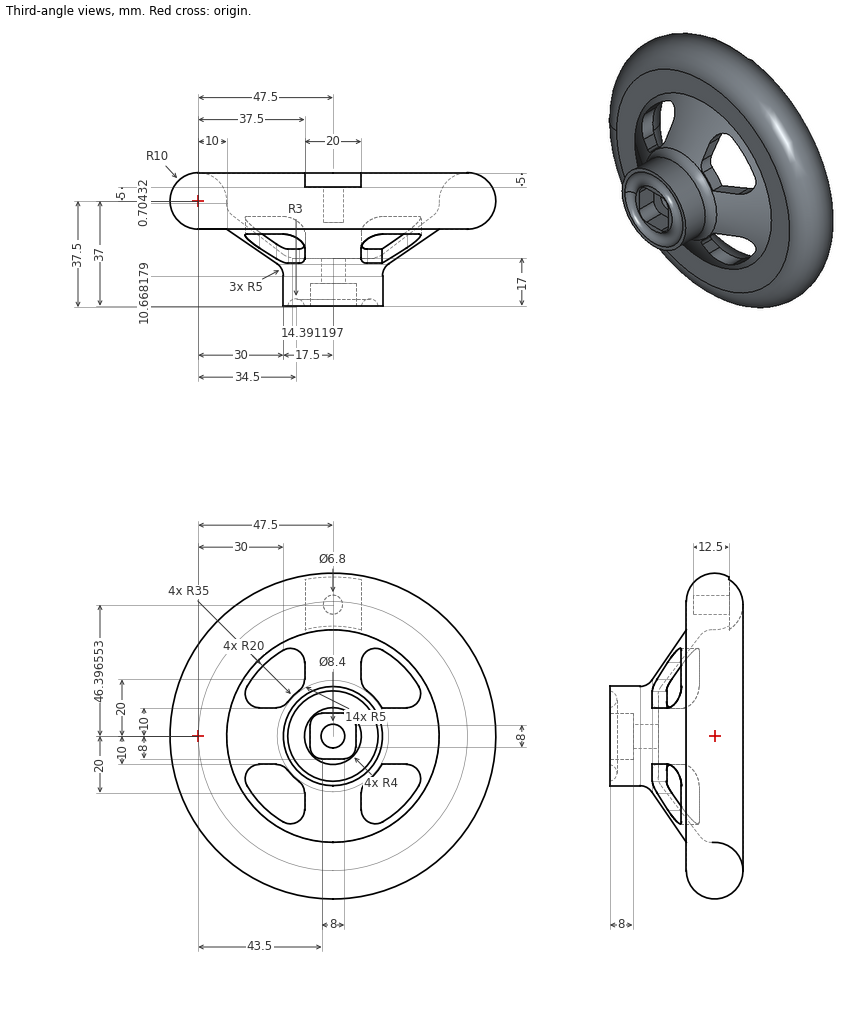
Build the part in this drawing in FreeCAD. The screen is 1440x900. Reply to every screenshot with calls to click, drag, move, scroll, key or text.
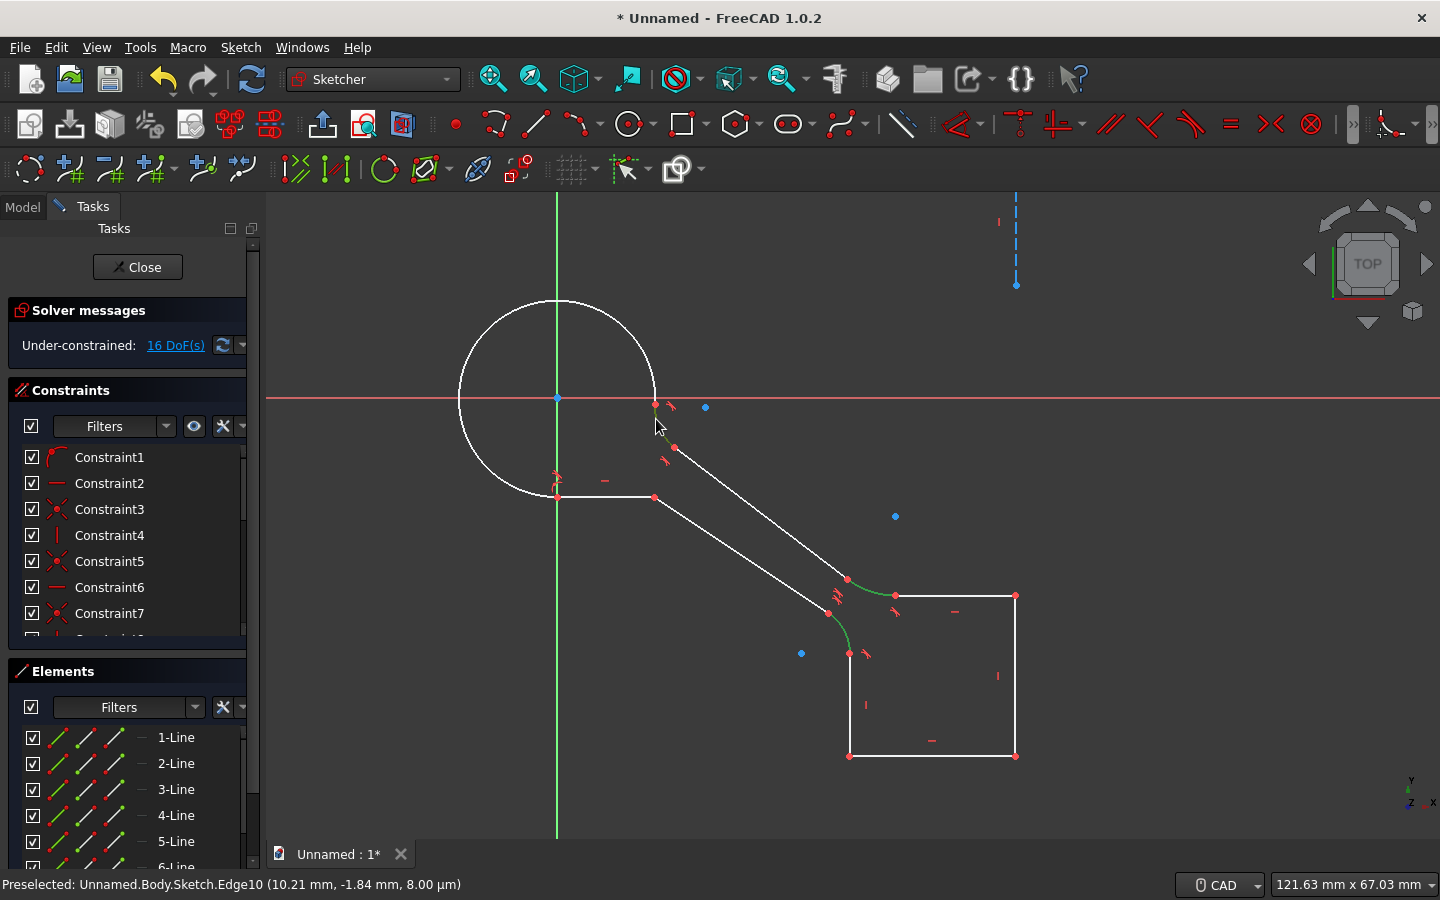
click(1232, 124)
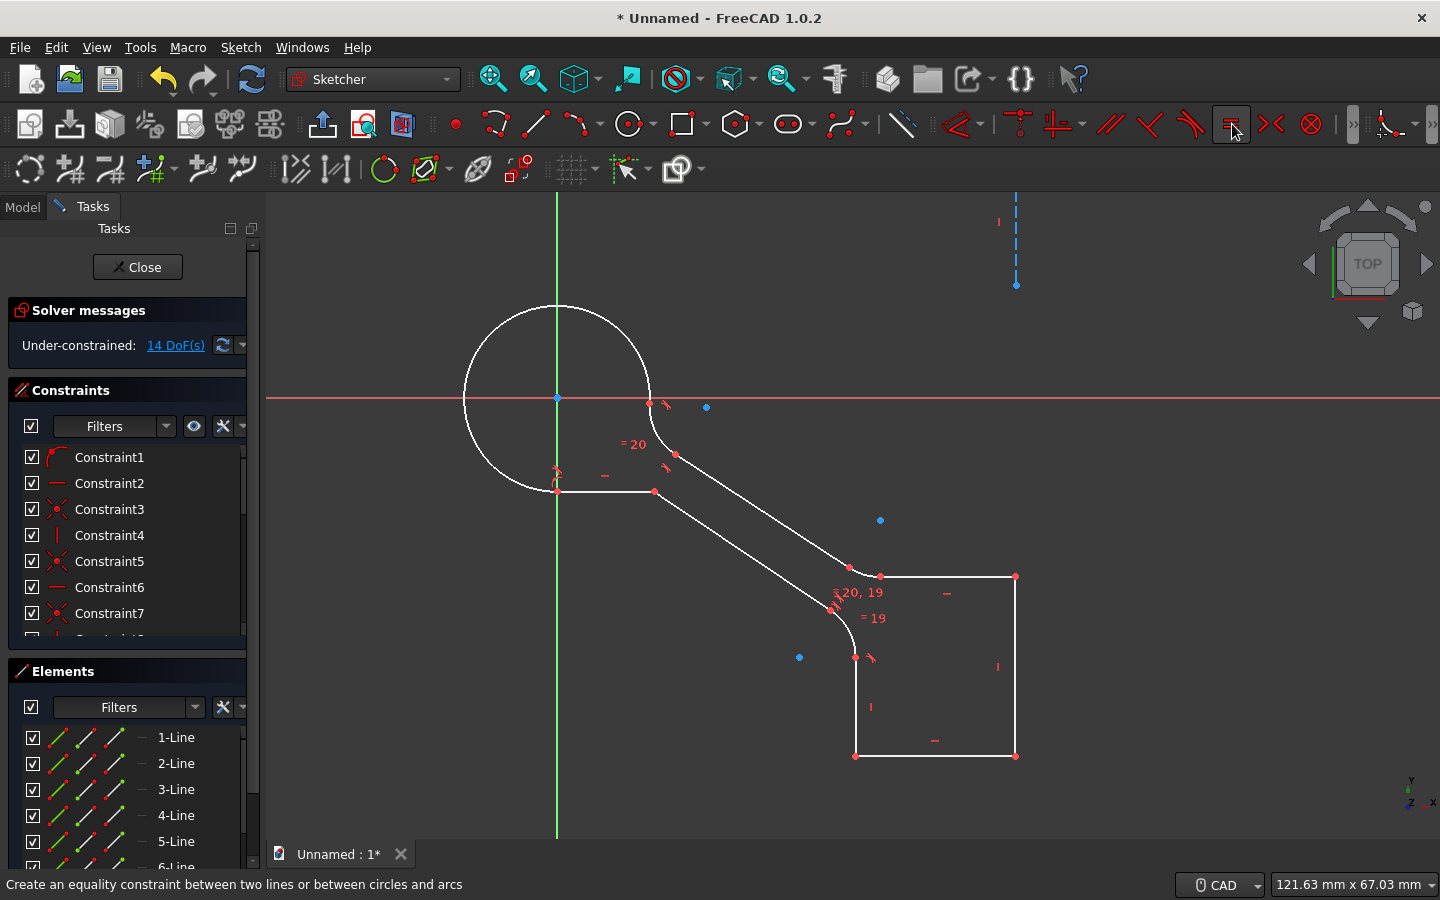
click(557, 399)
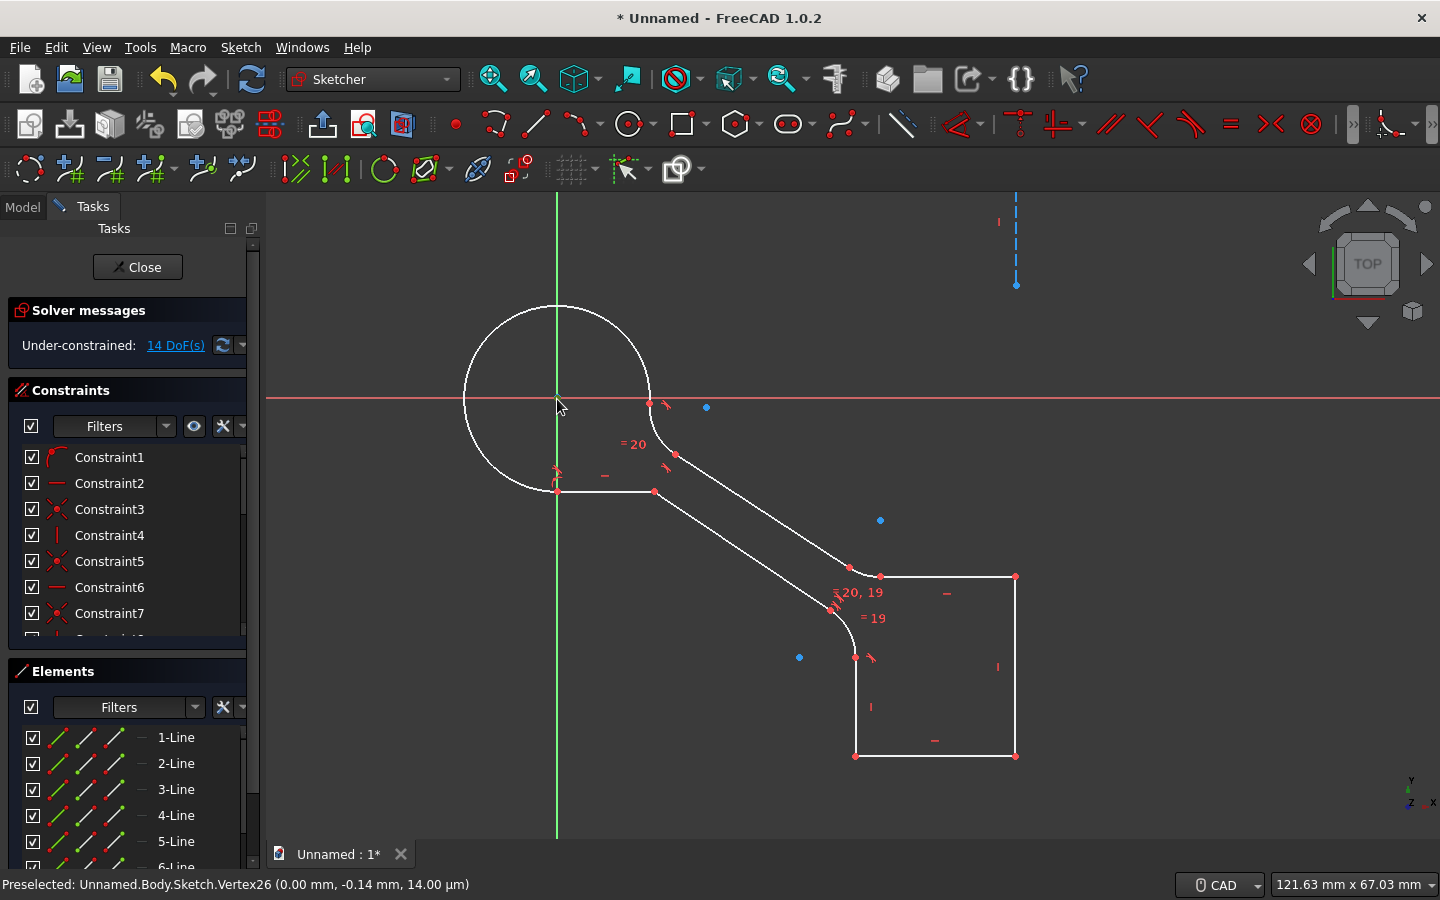
click(364, 398)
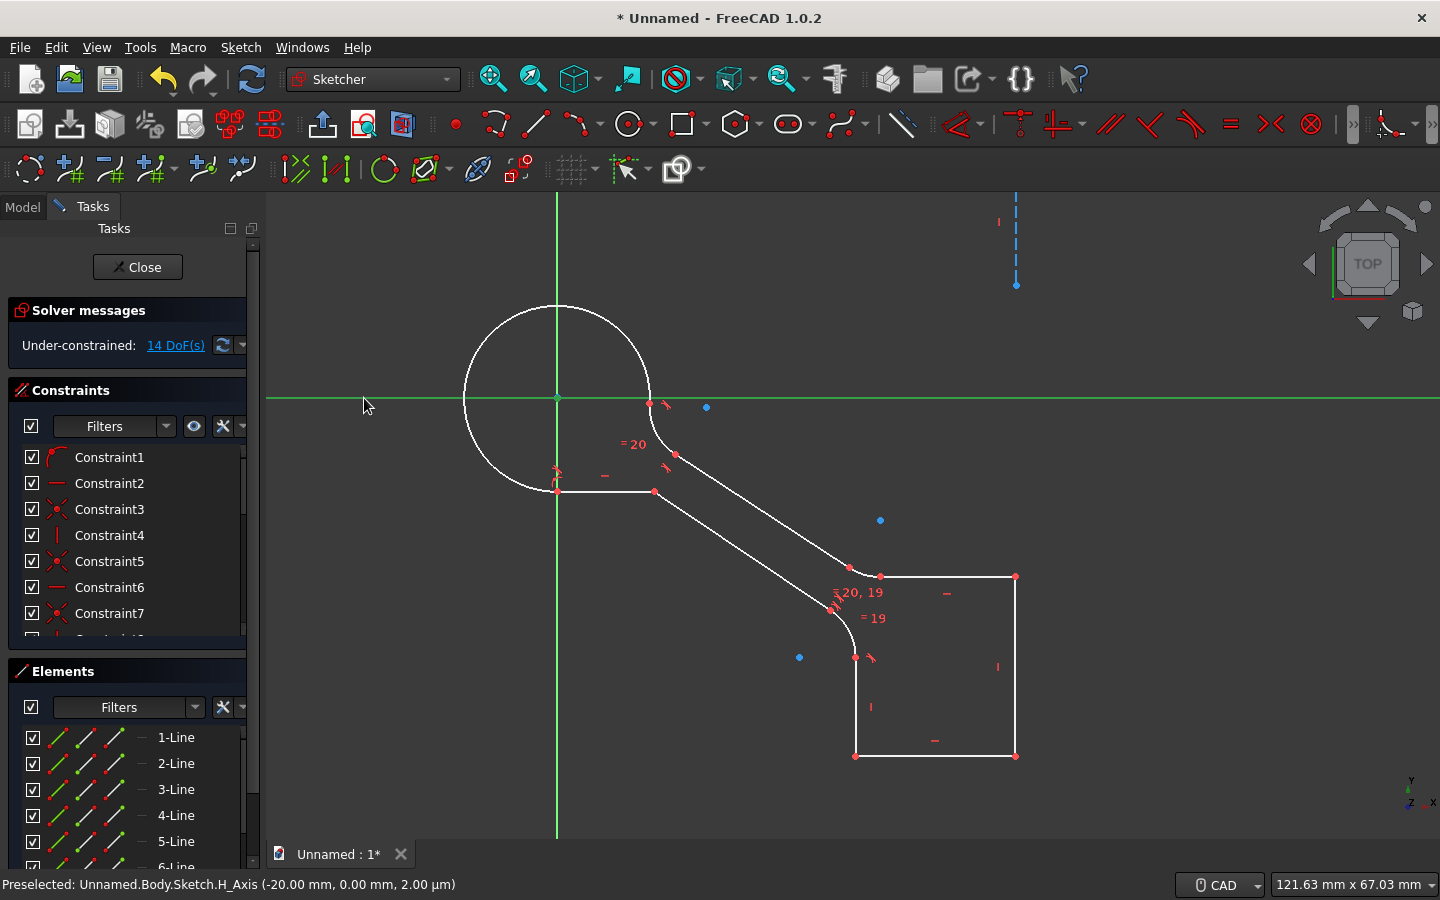
click(1018, 124)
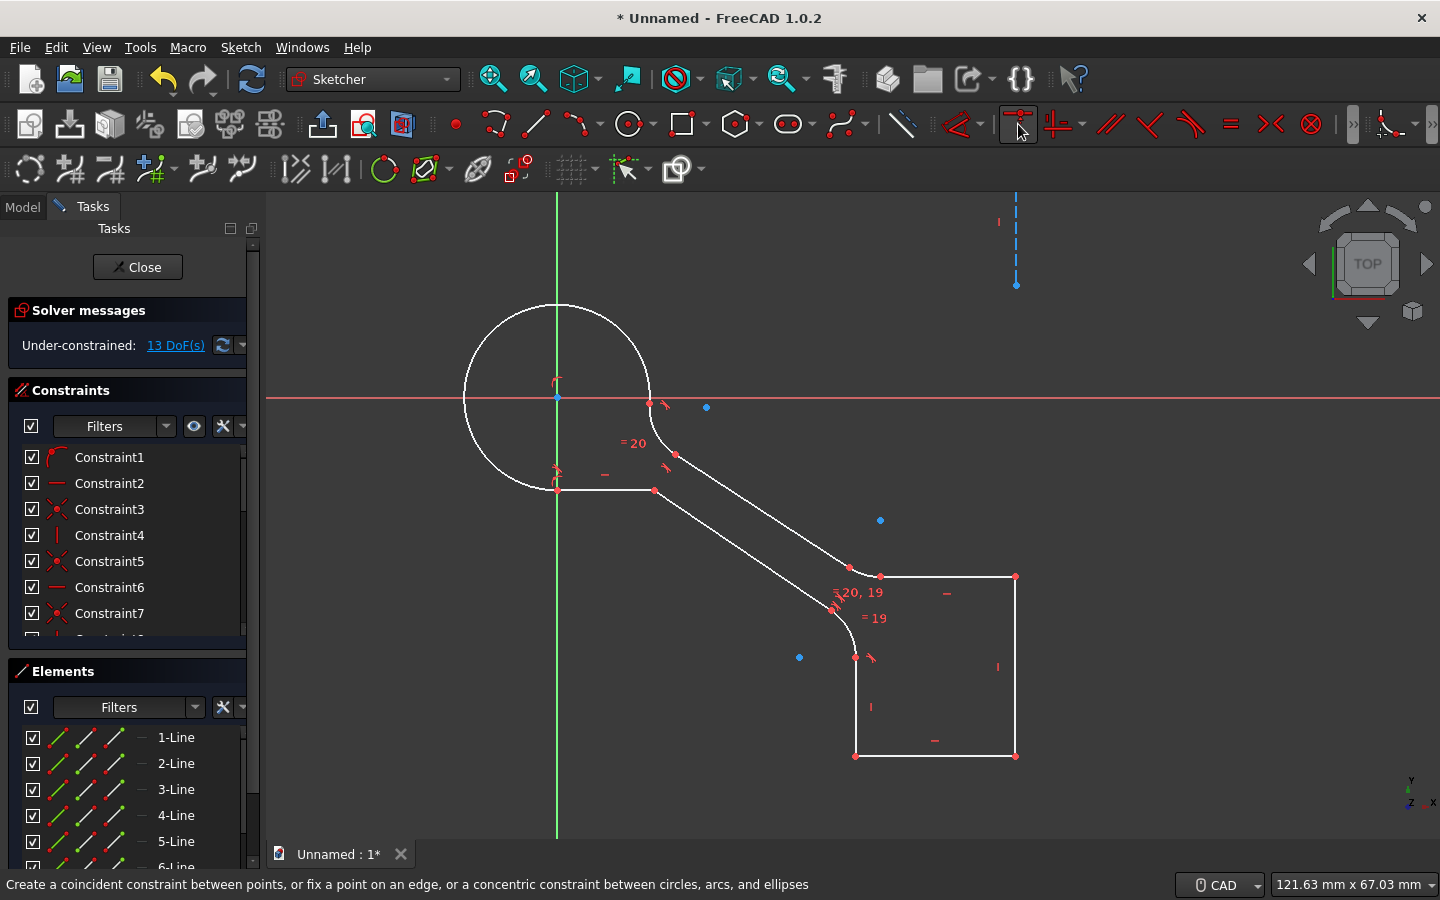
click(956, 124)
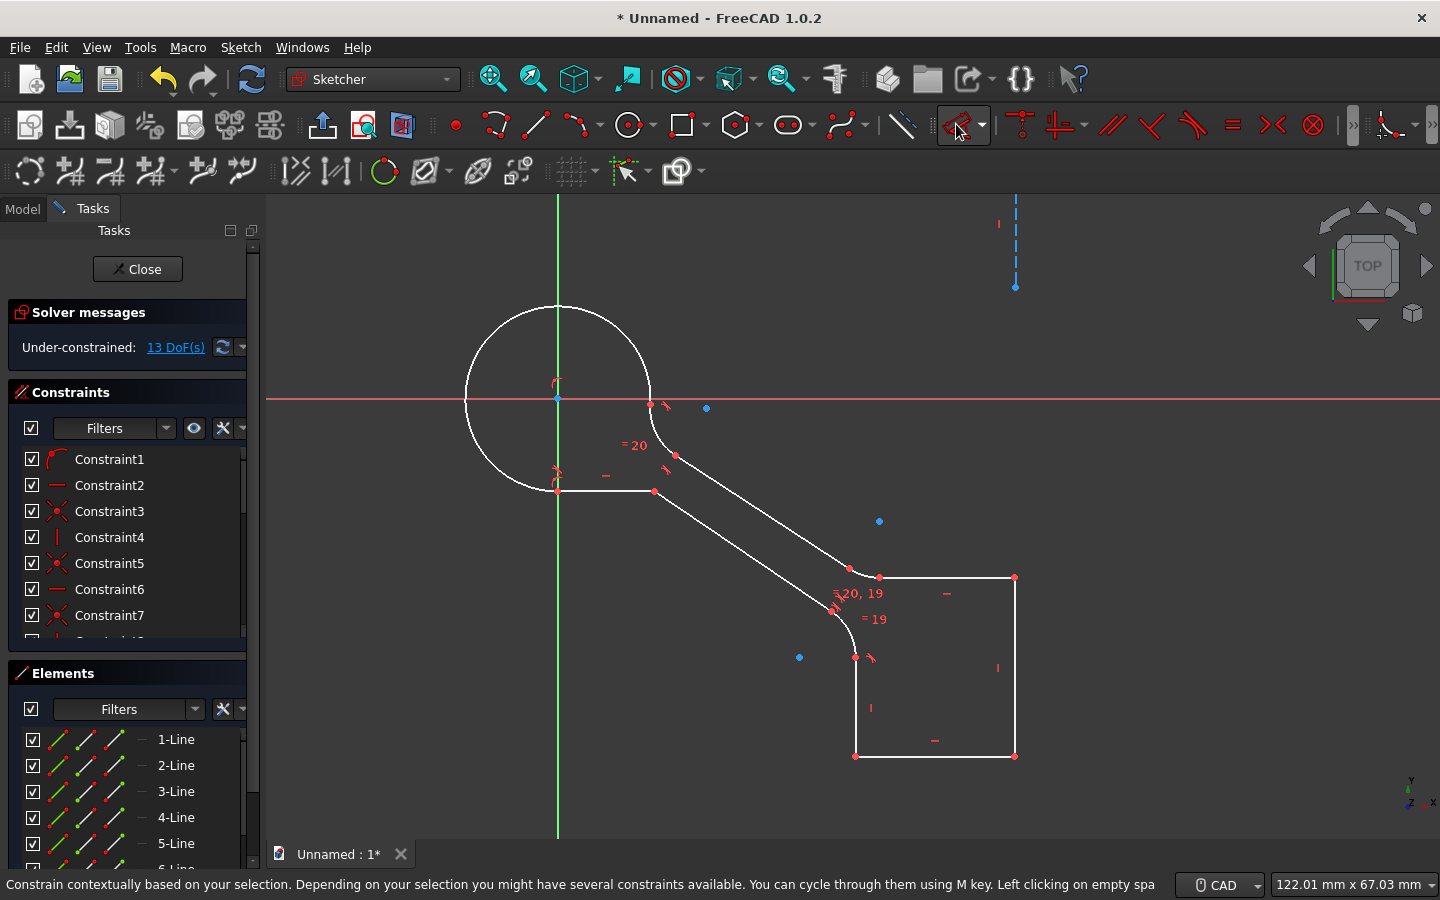
click(853, 642)
click(884, 633)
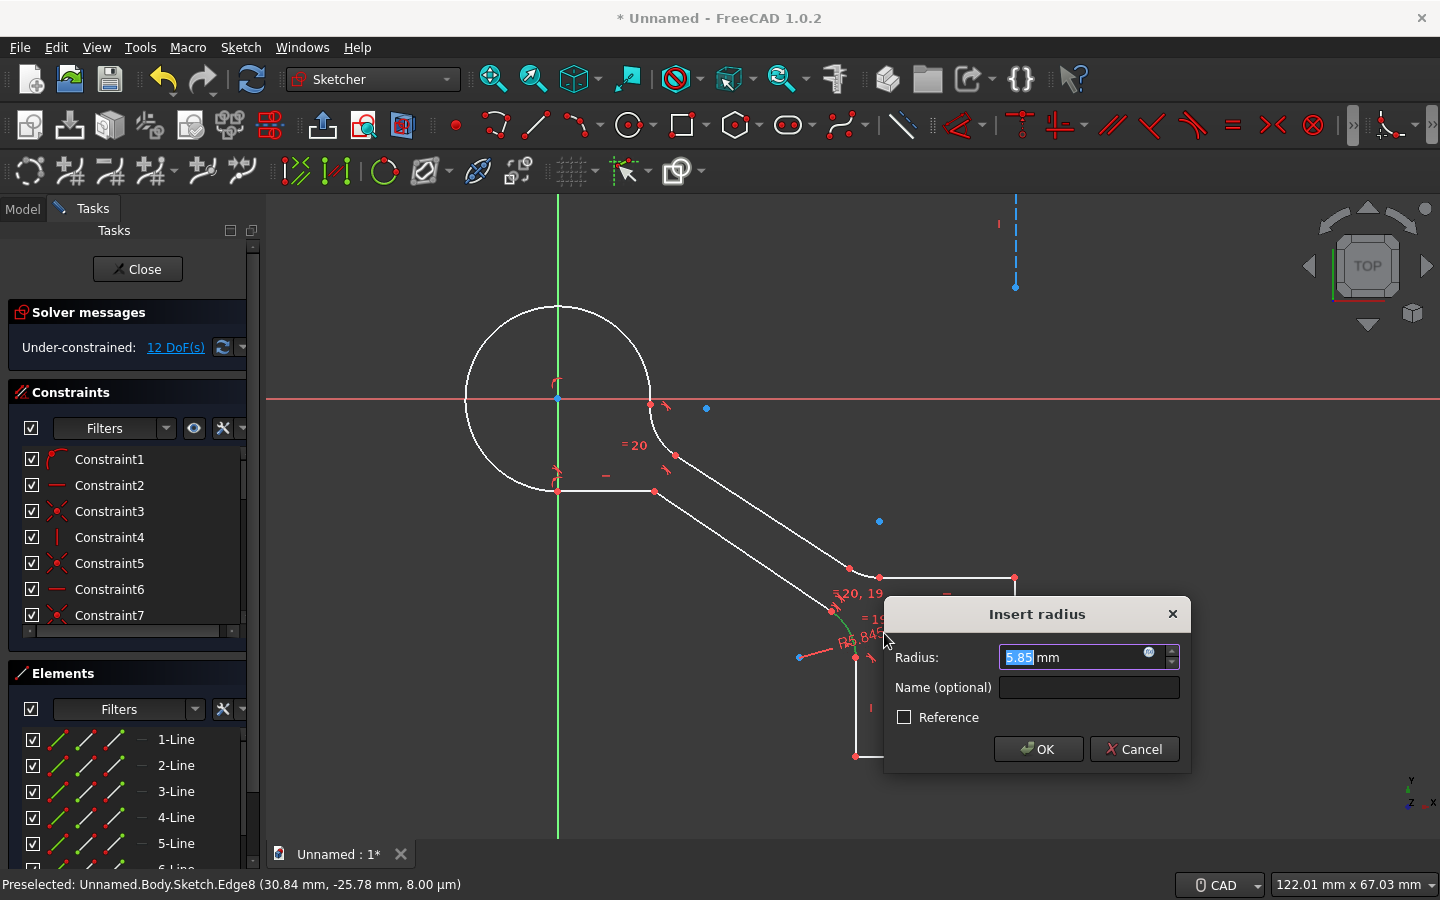
text(5)
key(Return)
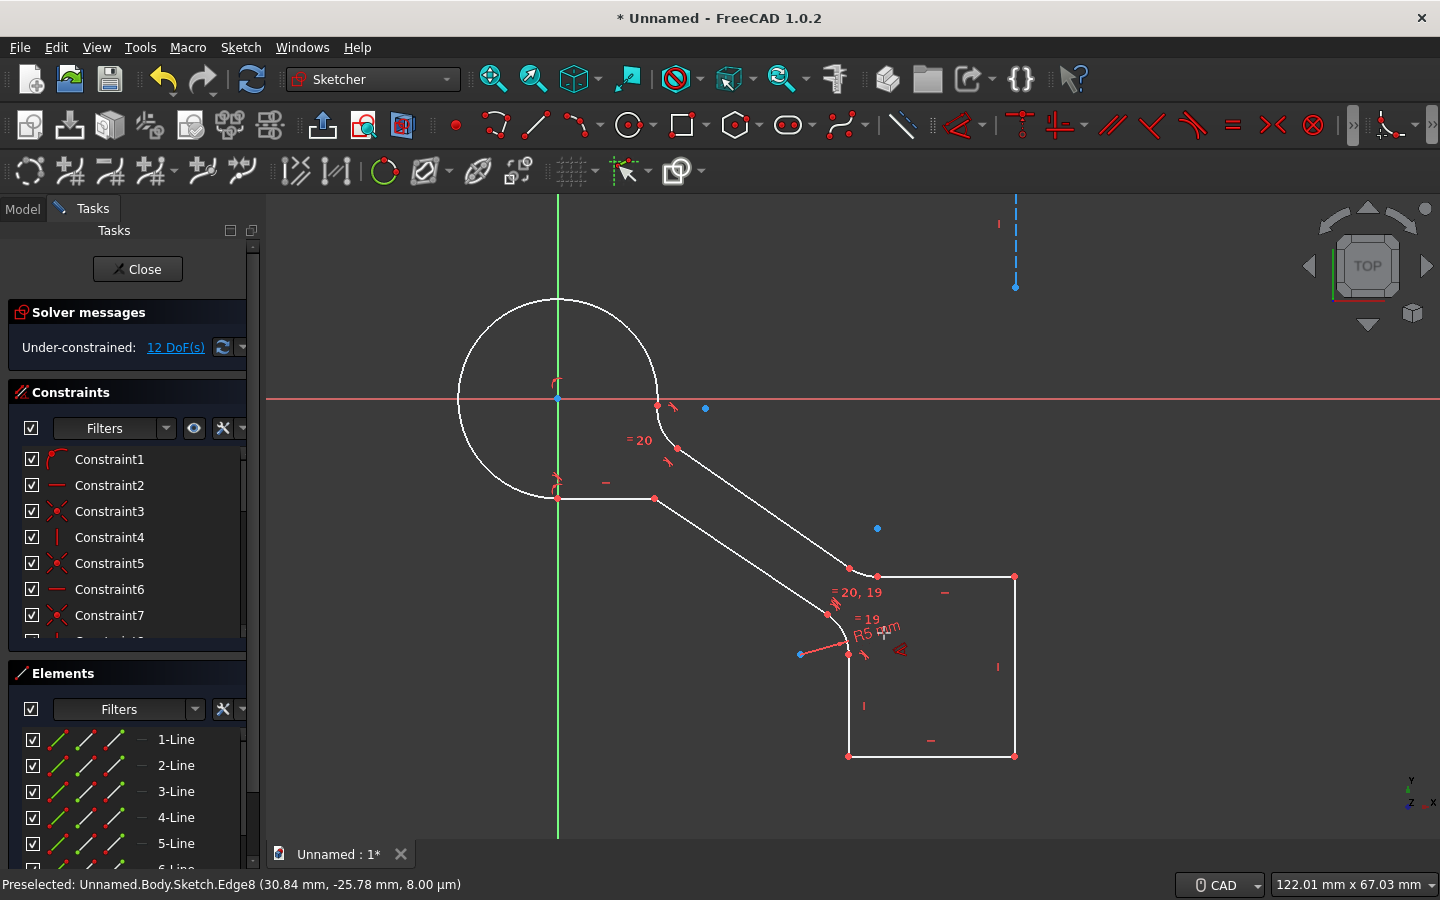
click(578, 301)
click(584, 270)